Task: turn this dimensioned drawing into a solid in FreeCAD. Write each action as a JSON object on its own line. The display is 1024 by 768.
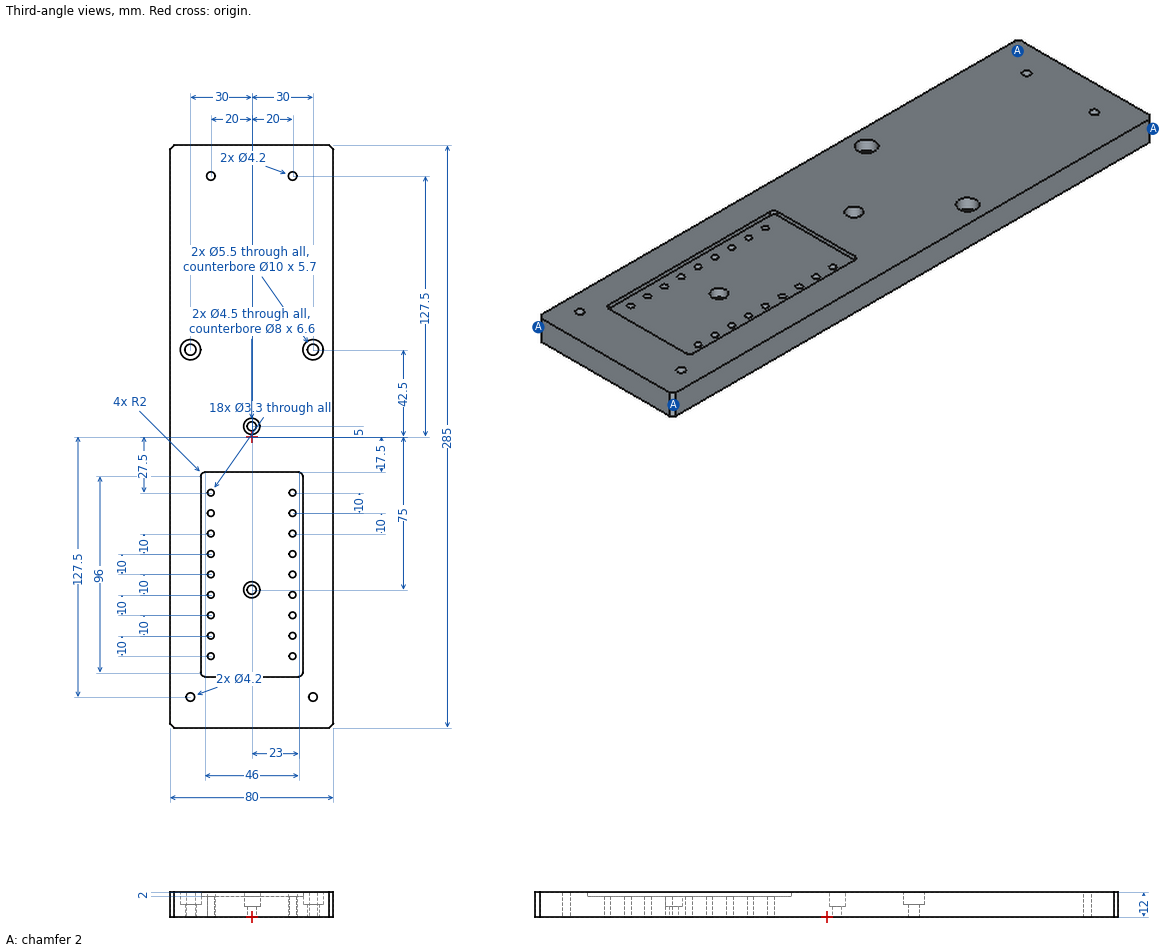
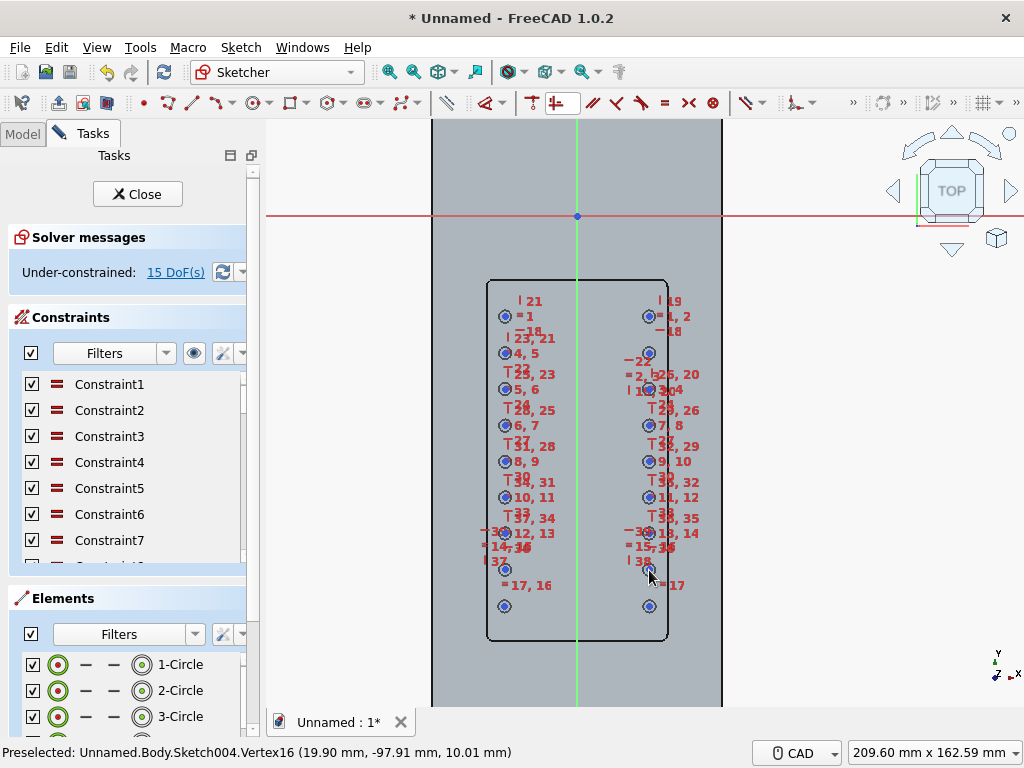
{"action": "left_click", "coordinate": [505, 570]}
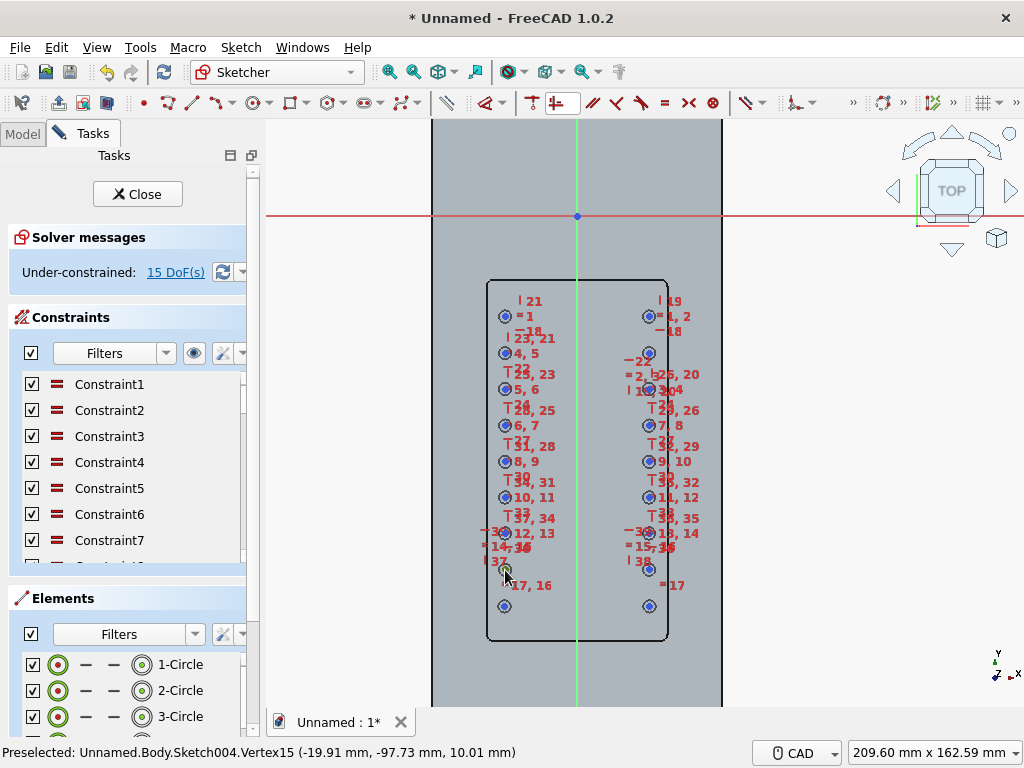
{"action": "left_click", "coordinate": [505, 606]}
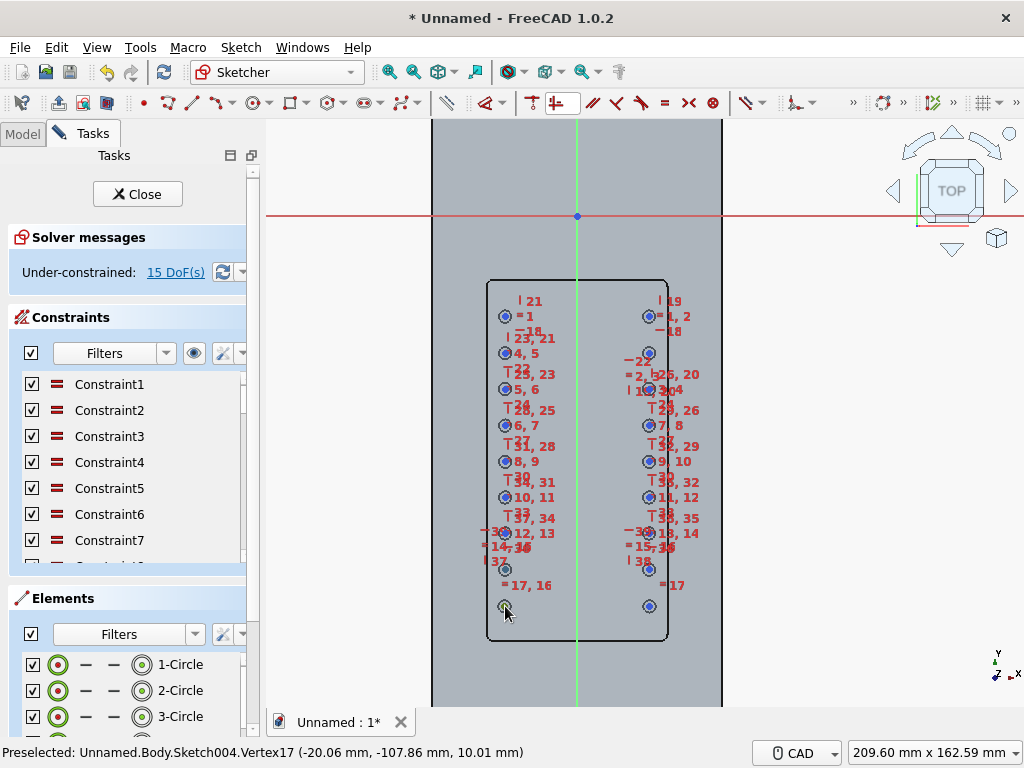
{"action": "key", "text": "v"}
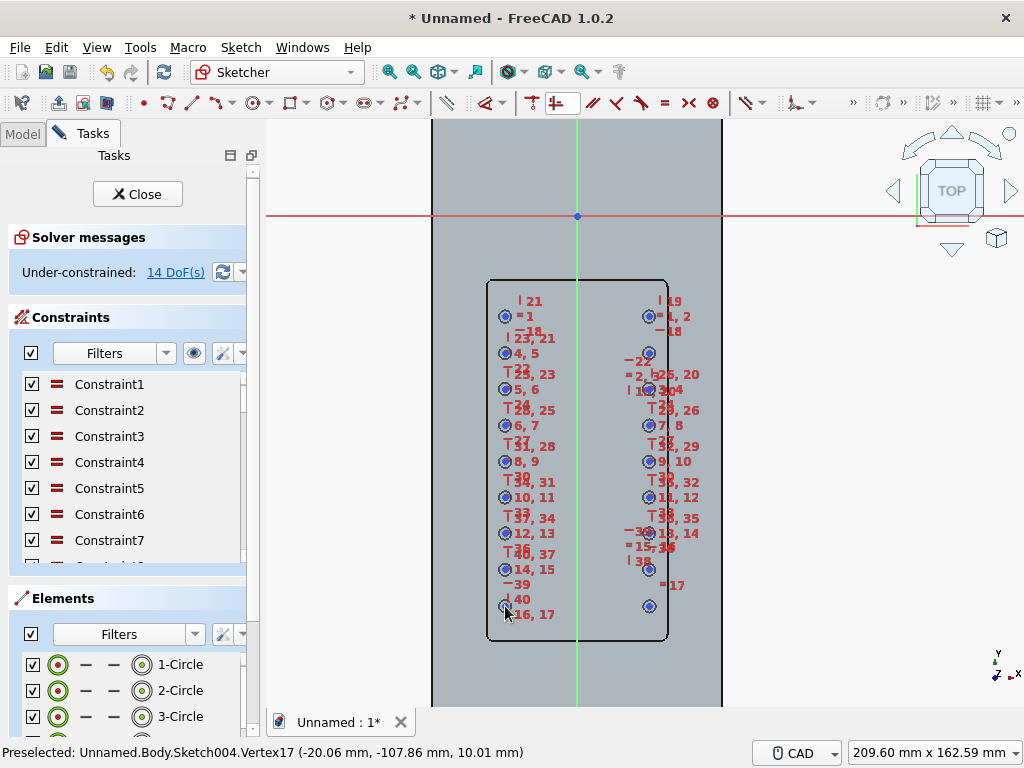
{"action": "left_click", "coordinate": [649, 570]}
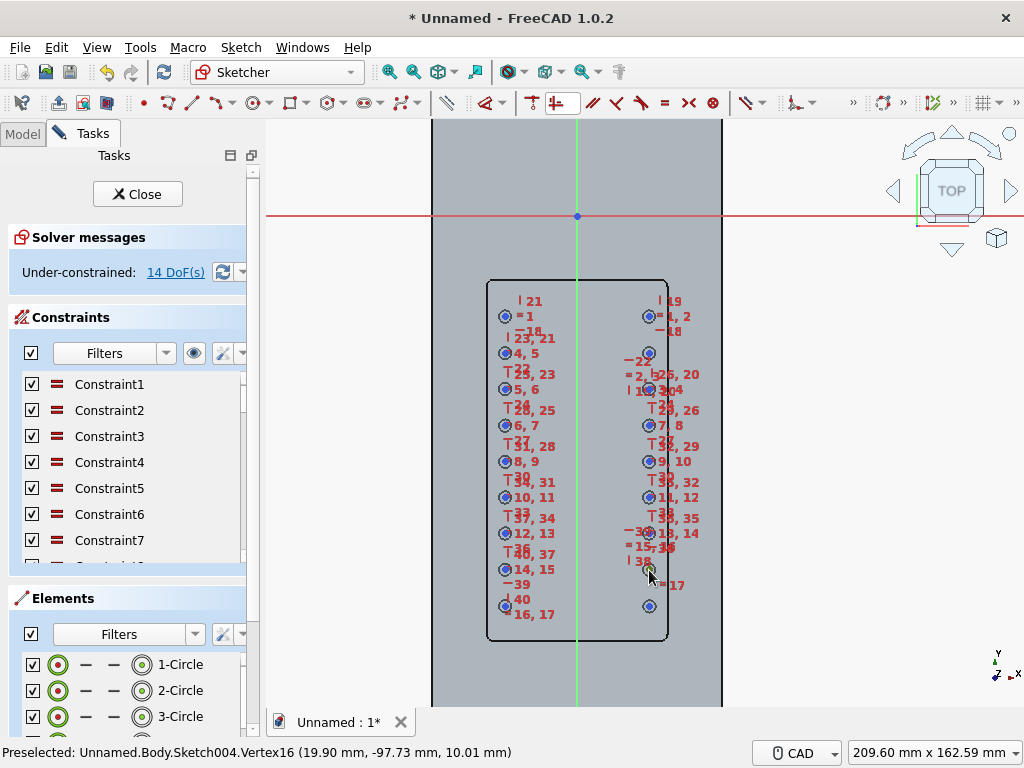
{"action": "left_click", "coordinate": [650, 606]}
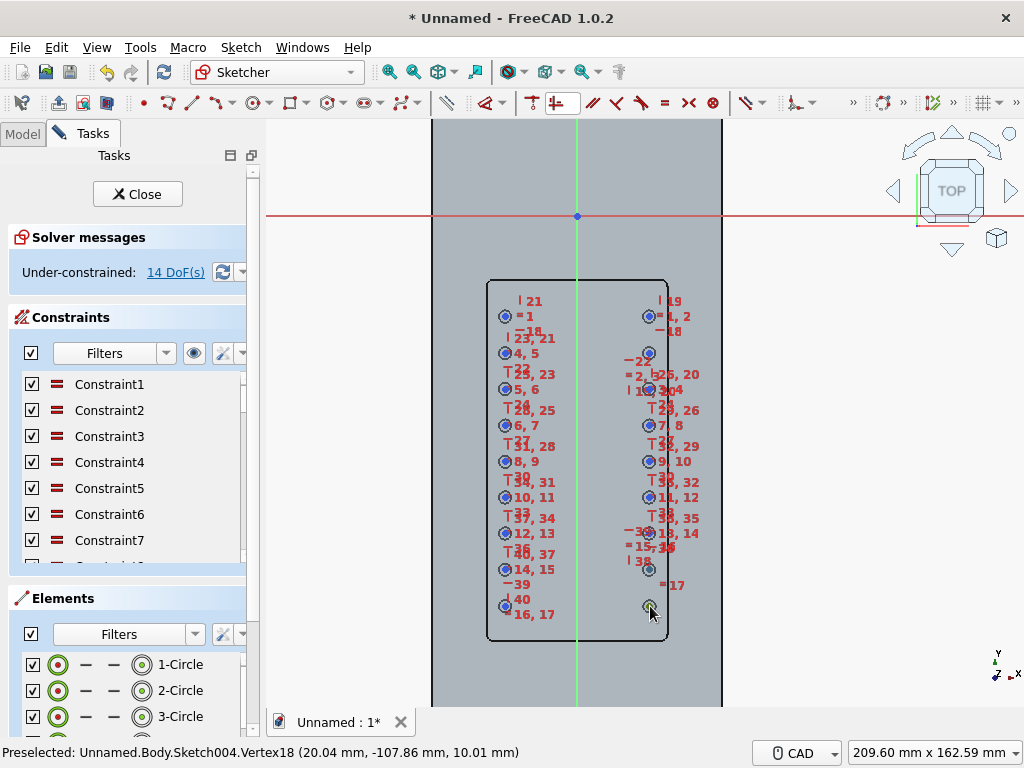
{"action": "key", "text": "v"}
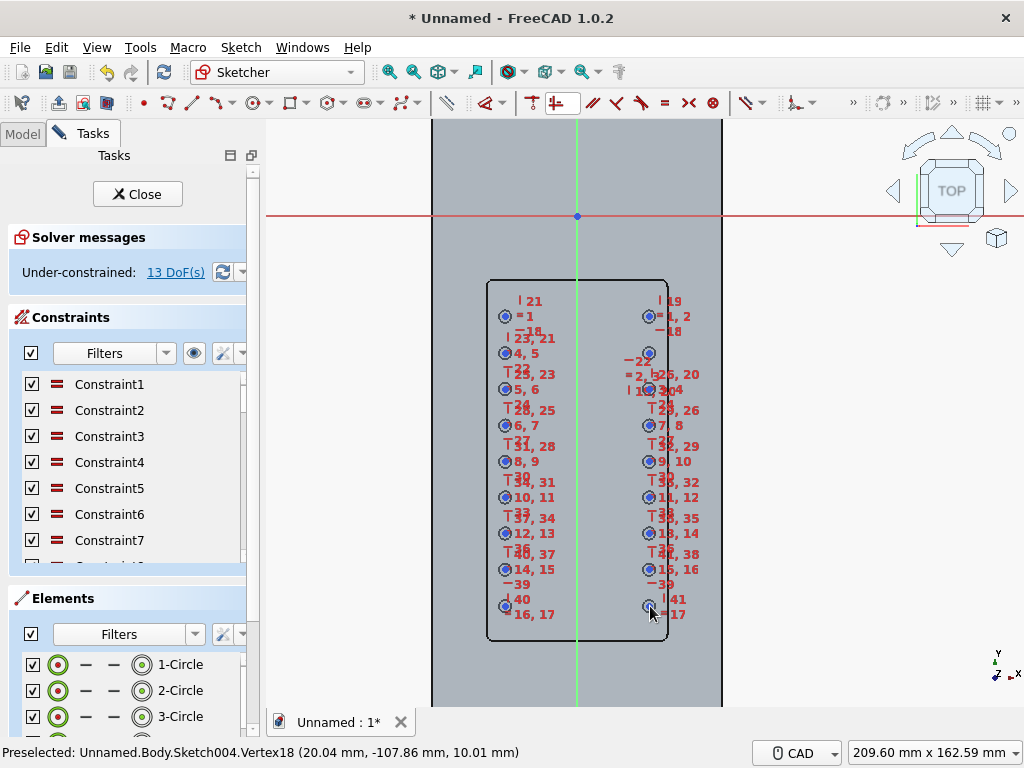
{"action": "scroll", "coordinate": [505, 606], "scroll_direction": "up", "scroll_amount": 4}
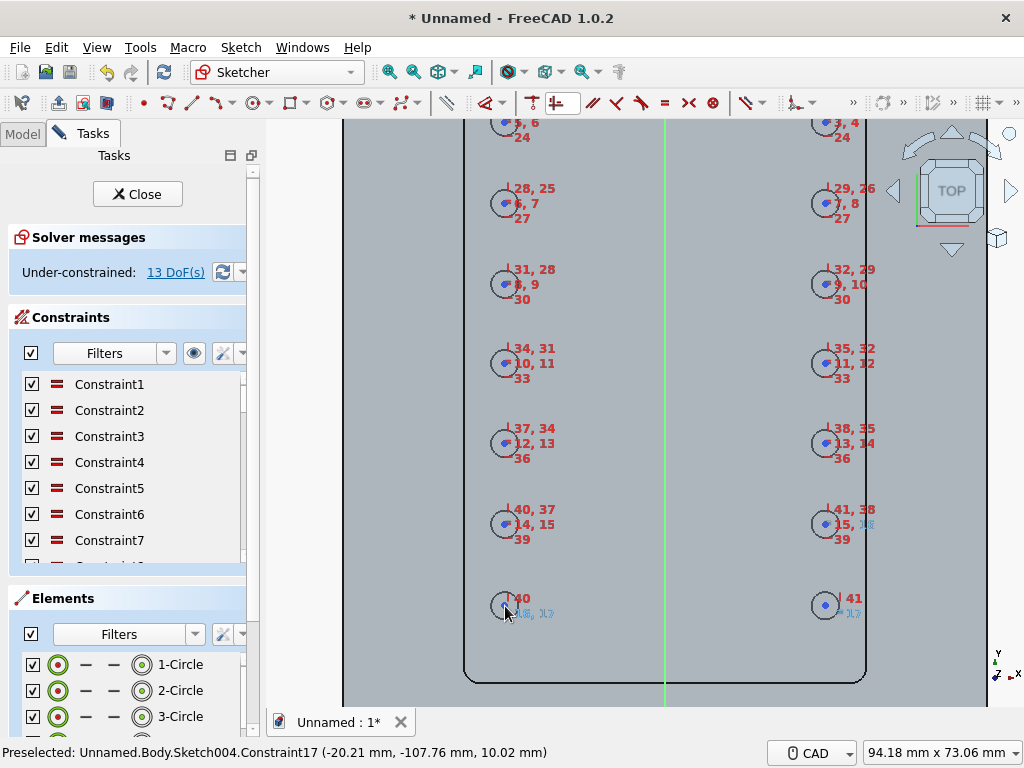
{"action": "scroll", "coordinate": [505, 606], "scroll_direction": "up", "scroll_amount": 4}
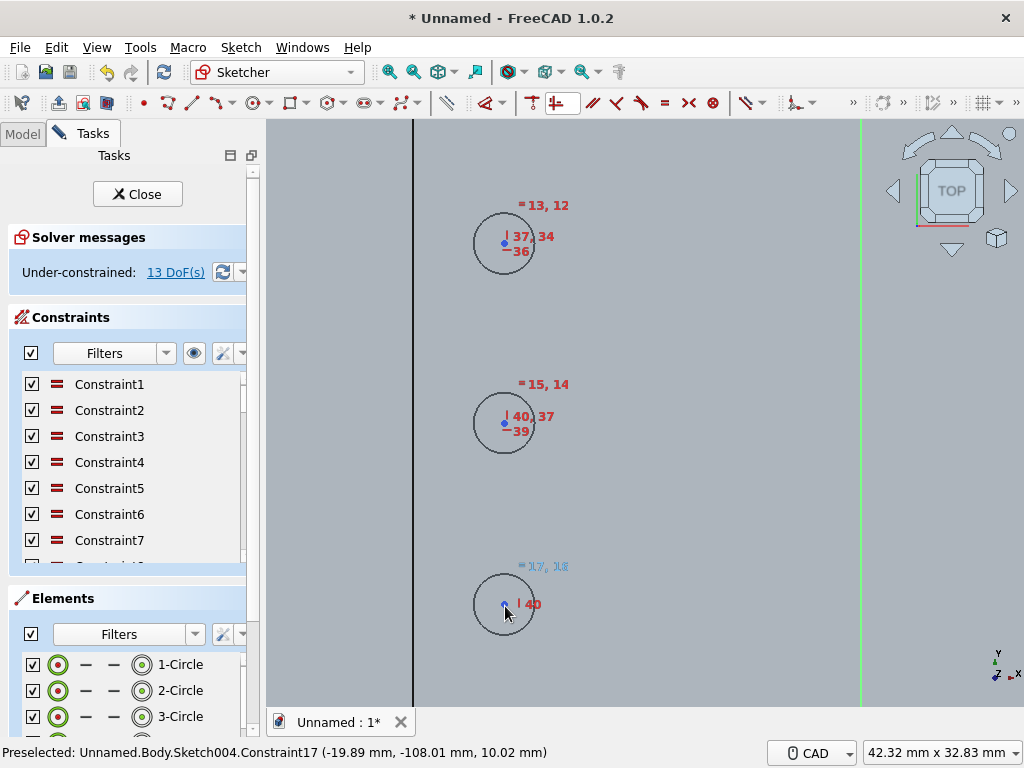
{"action": "left_click", "coordinate": [504, 605]}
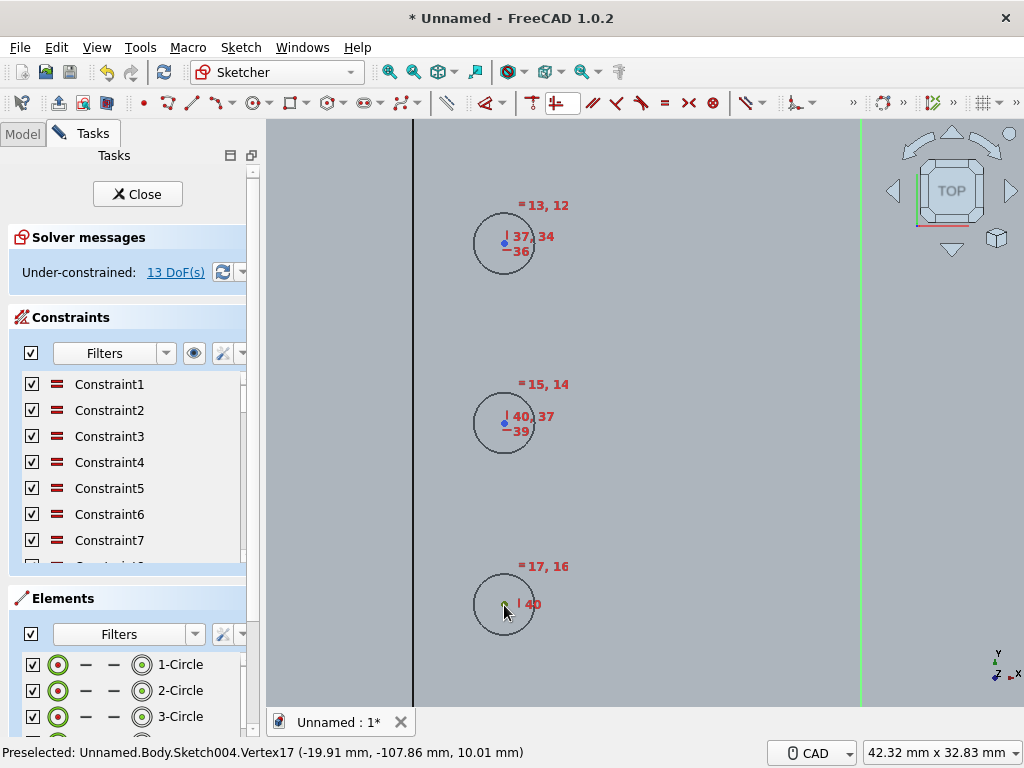
{"action": "scroll", "coordinate": [505, 606], "scroll_direction": "down", "scroll_amount": 8}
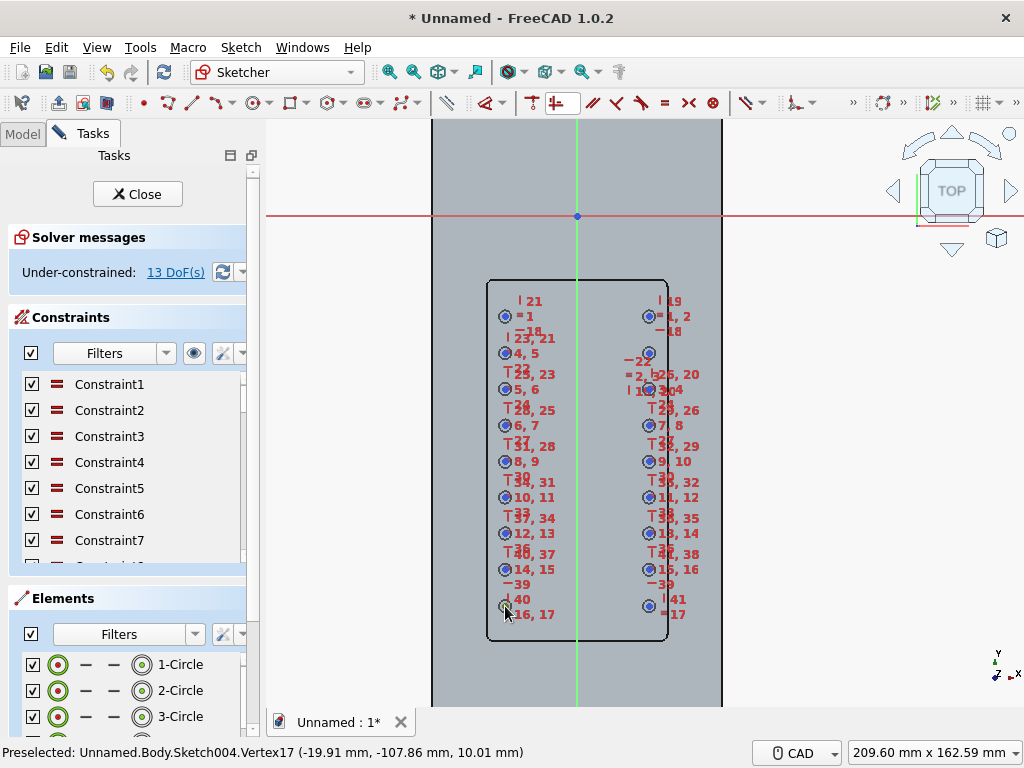
{"action": "left_click", "coordinate": [649, 606]}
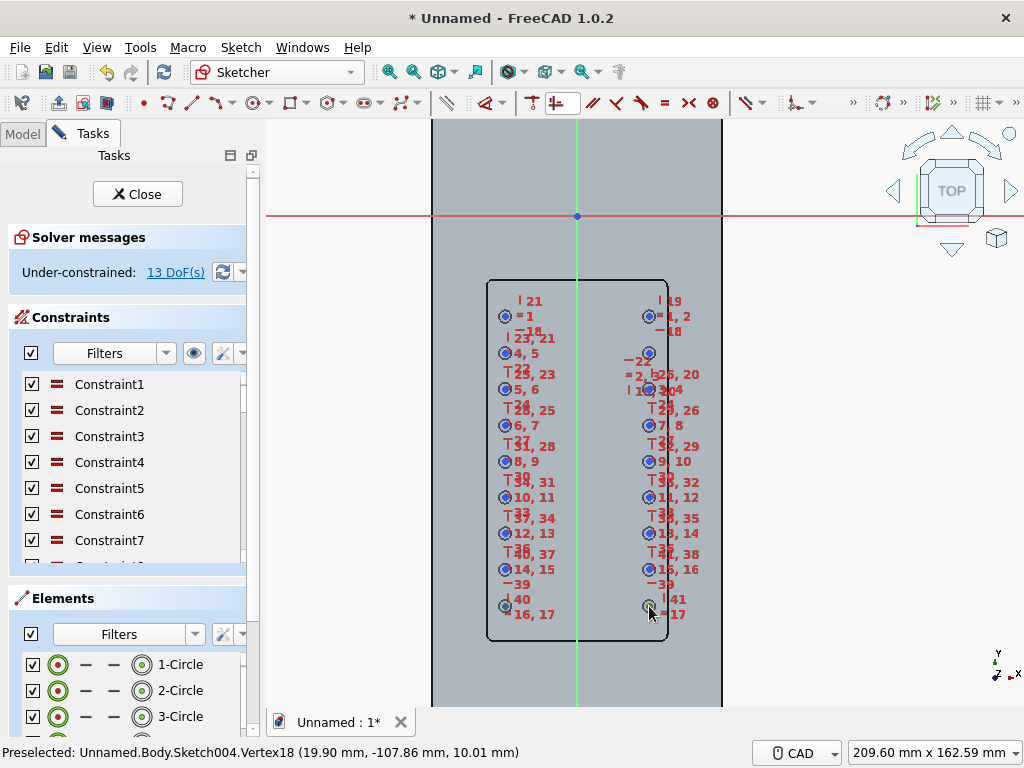
{"action": "key", "text": "h"}